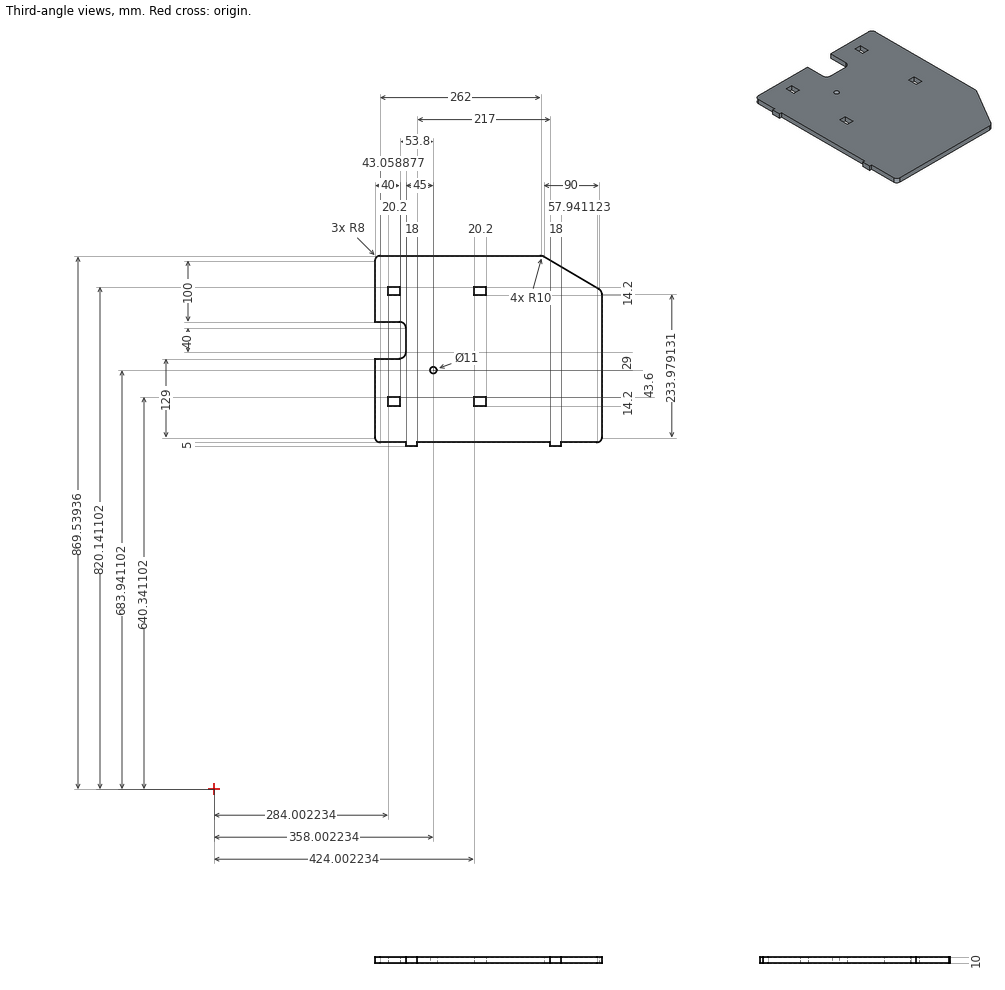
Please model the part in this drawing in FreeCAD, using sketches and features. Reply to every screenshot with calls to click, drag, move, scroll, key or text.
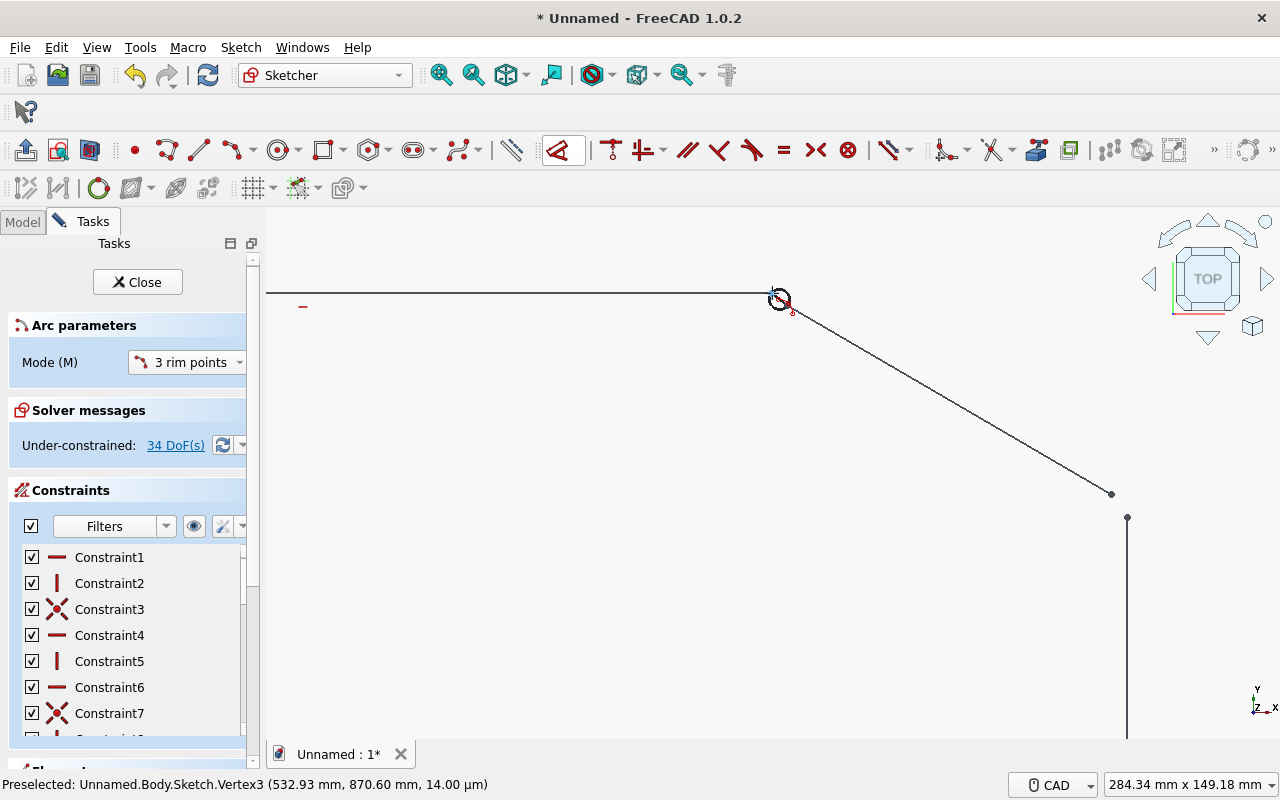
scroll(781, 293, up, 13)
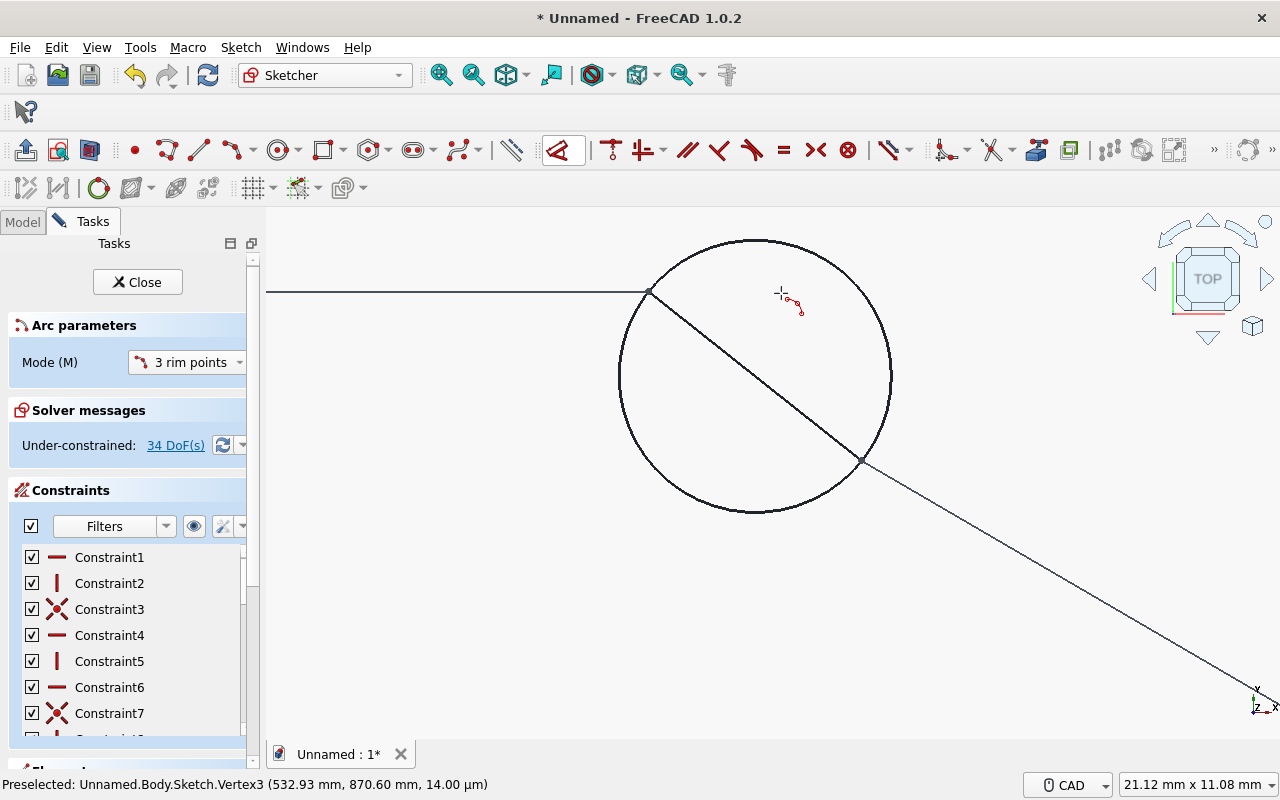
click(779, 292)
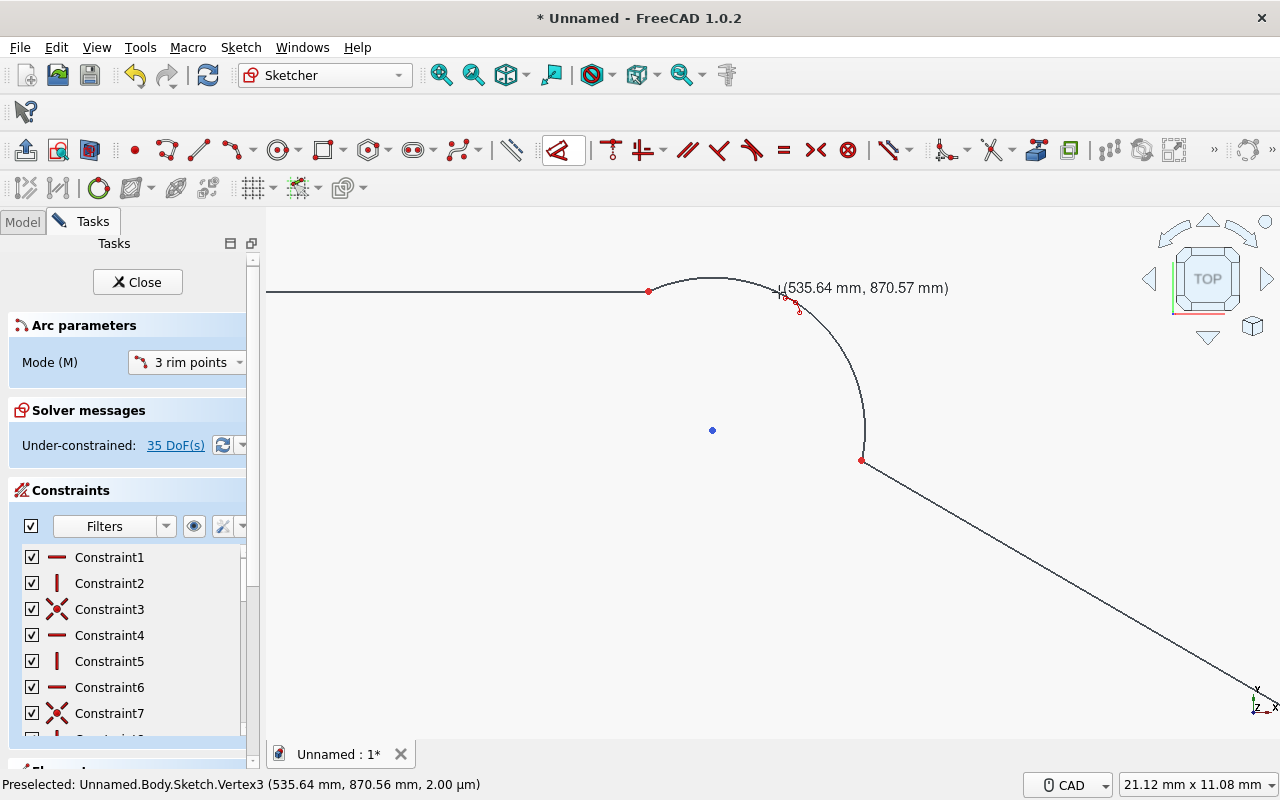
scroll(704, 473, down, 15)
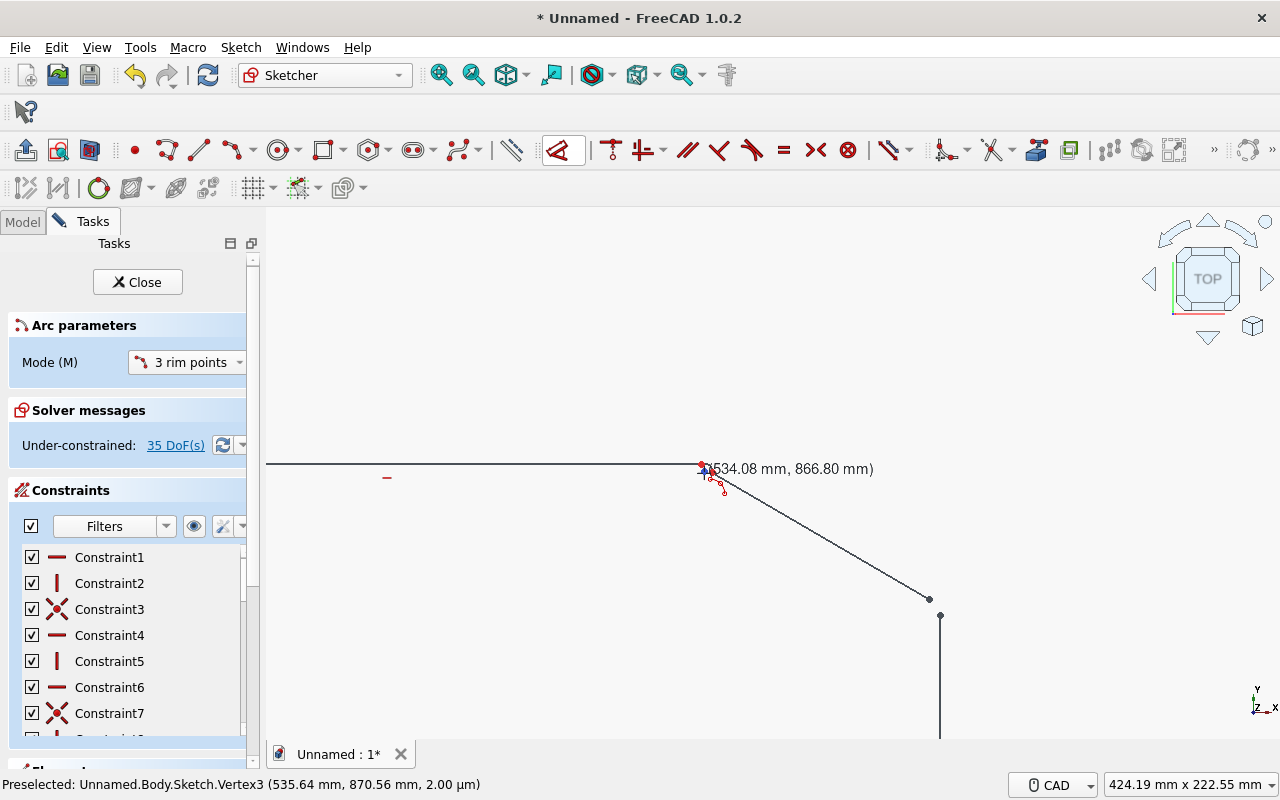
scroll(808, 269, down, 9)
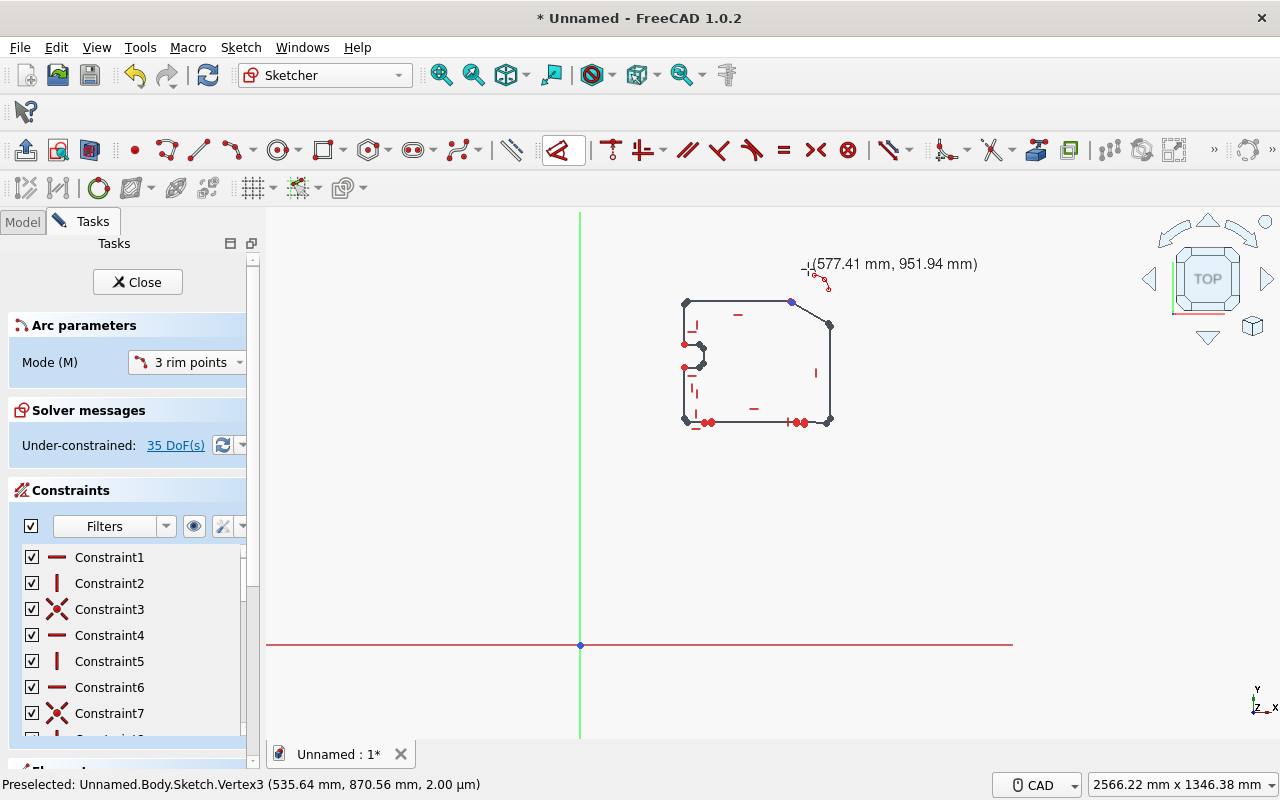
scroll(687, 301, up, 7)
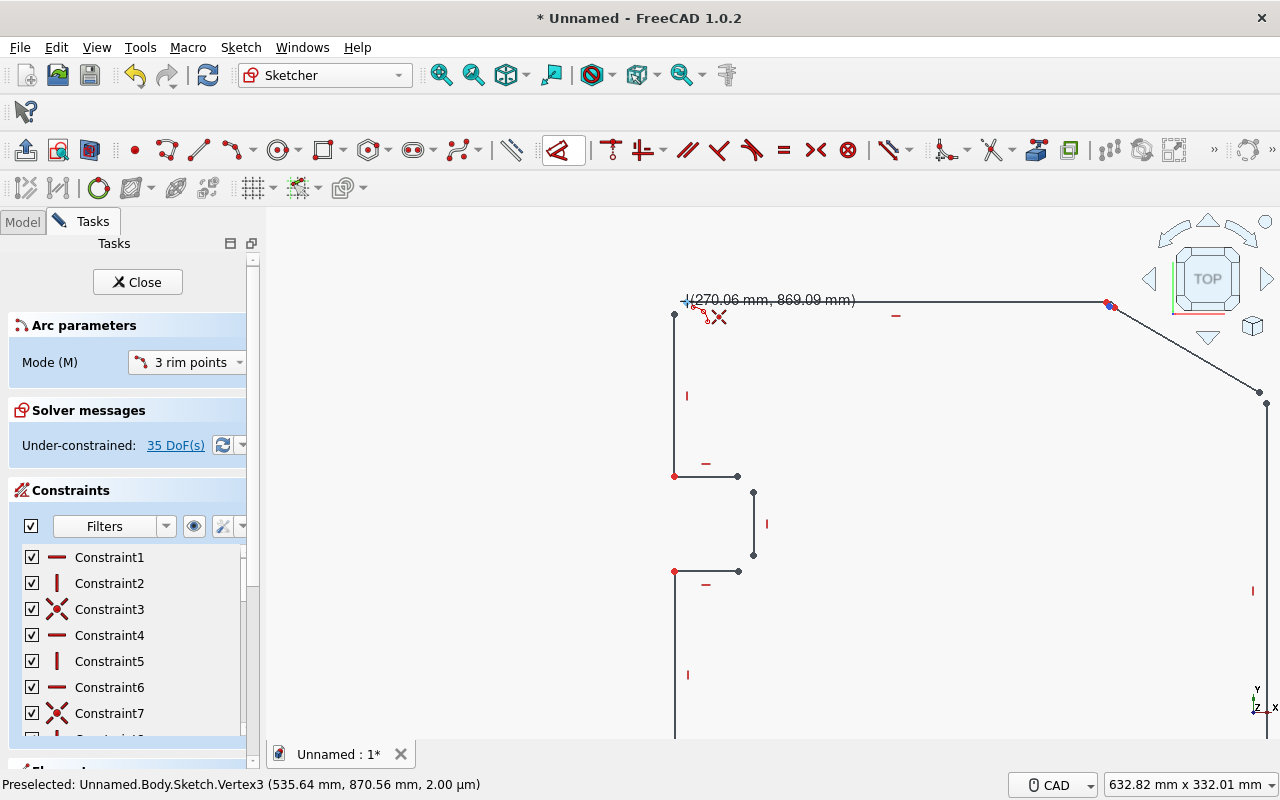
click(686, 302)
click(674, 315)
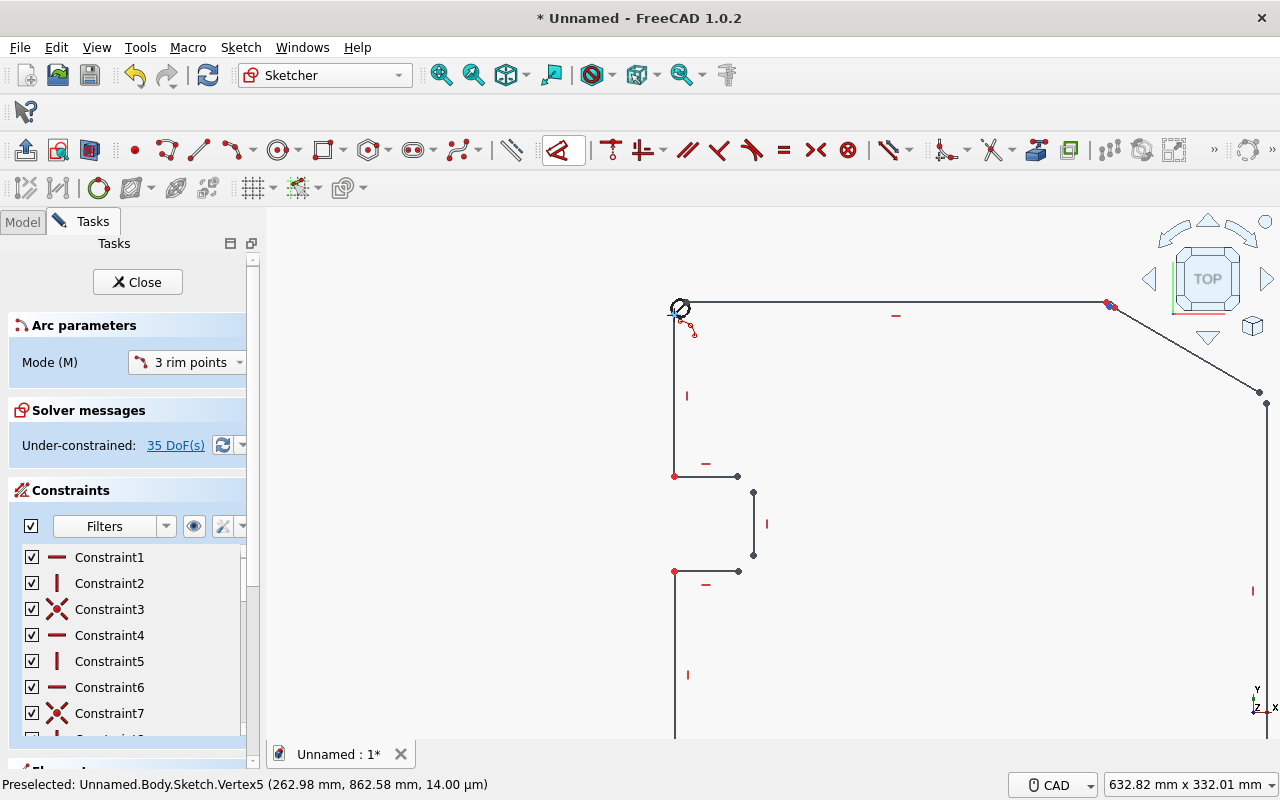
scroll(678, 305, up, 8)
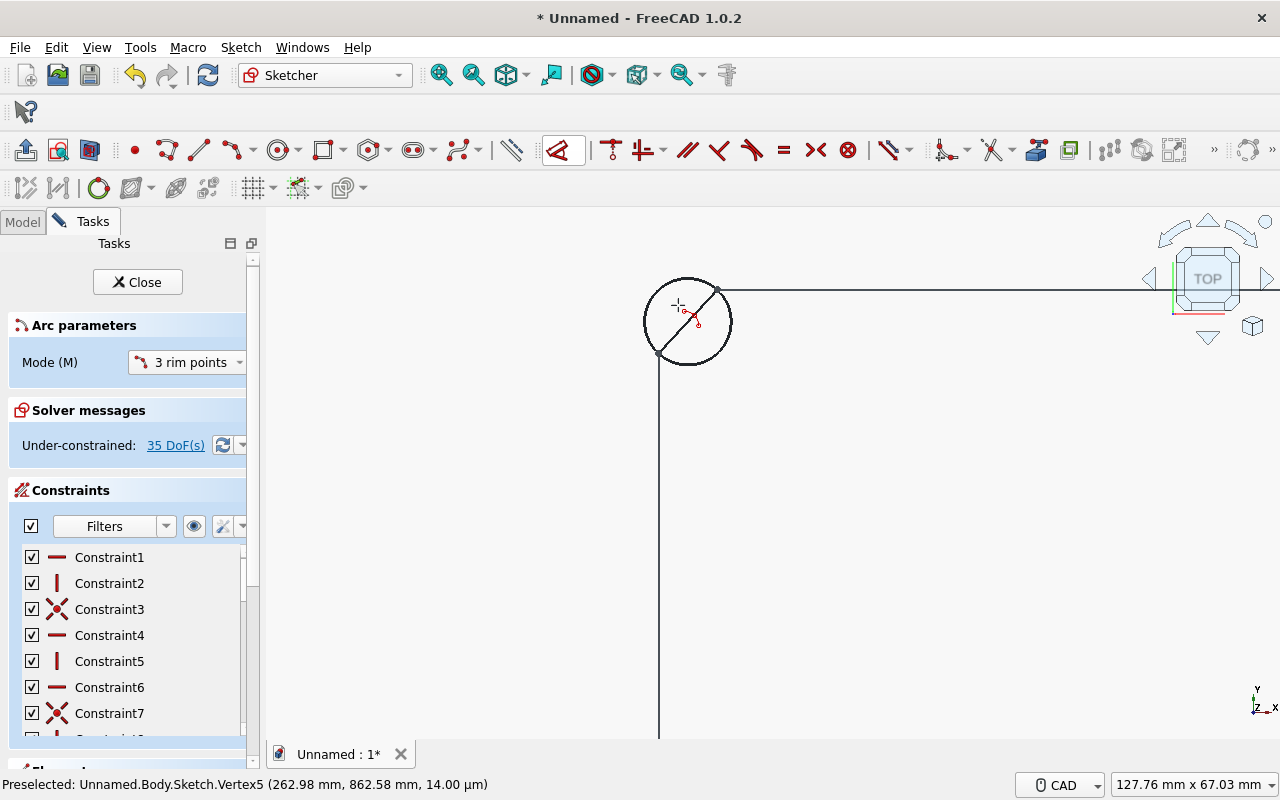
click(677, 306)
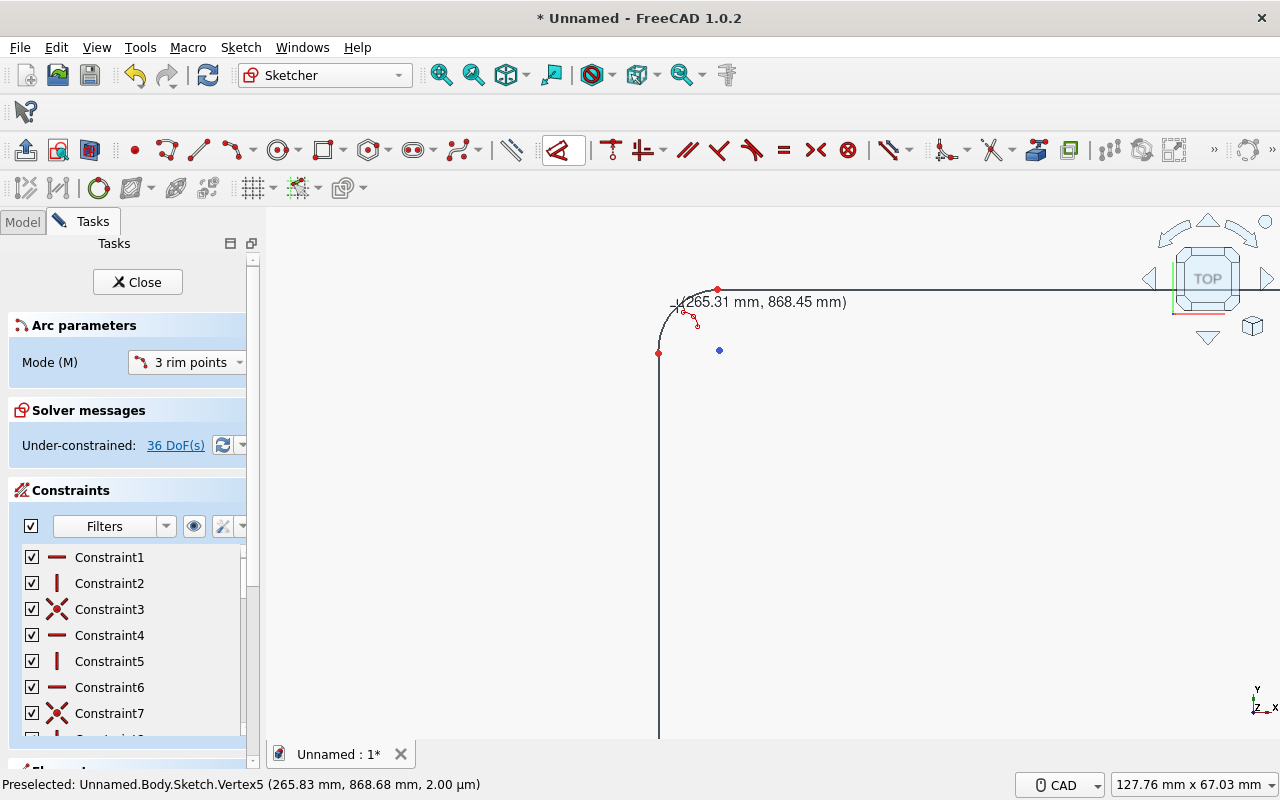
scroll(685, 302, down, 15)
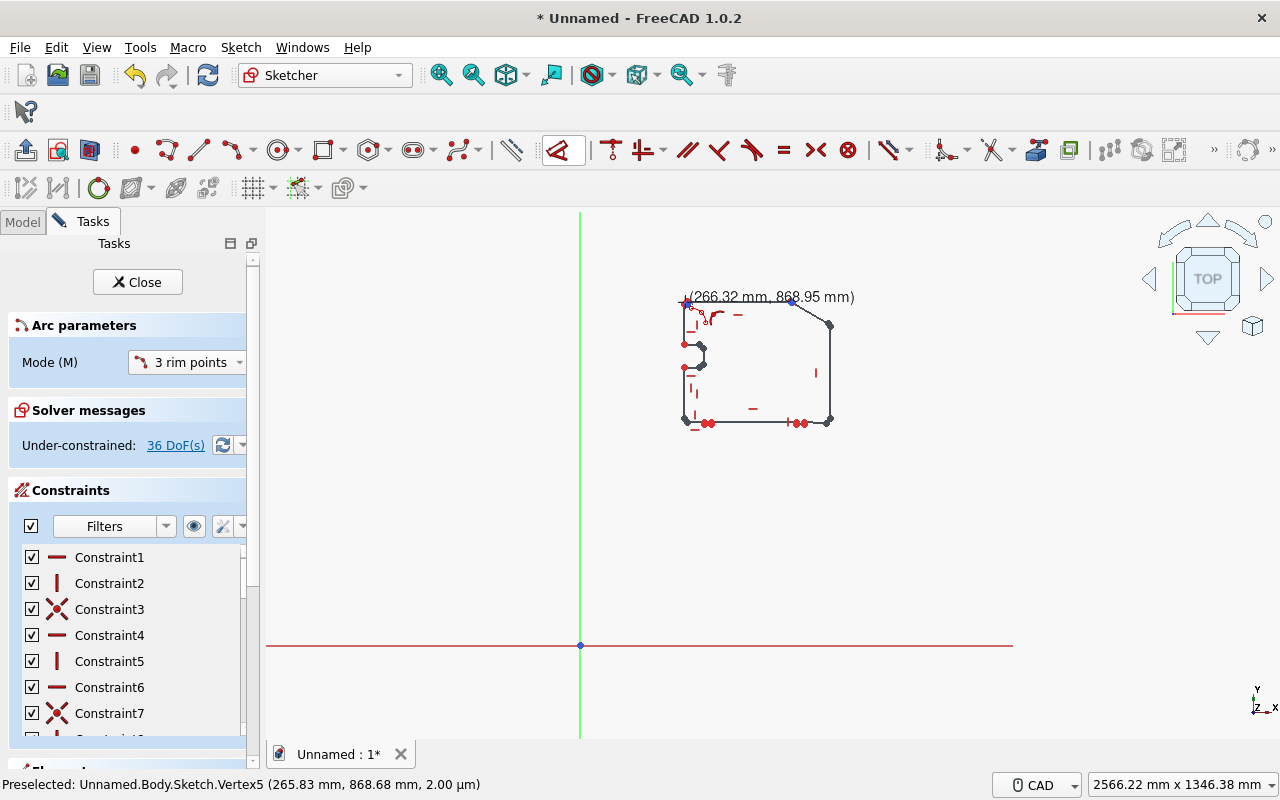
scroll(700, 344, up, 6)